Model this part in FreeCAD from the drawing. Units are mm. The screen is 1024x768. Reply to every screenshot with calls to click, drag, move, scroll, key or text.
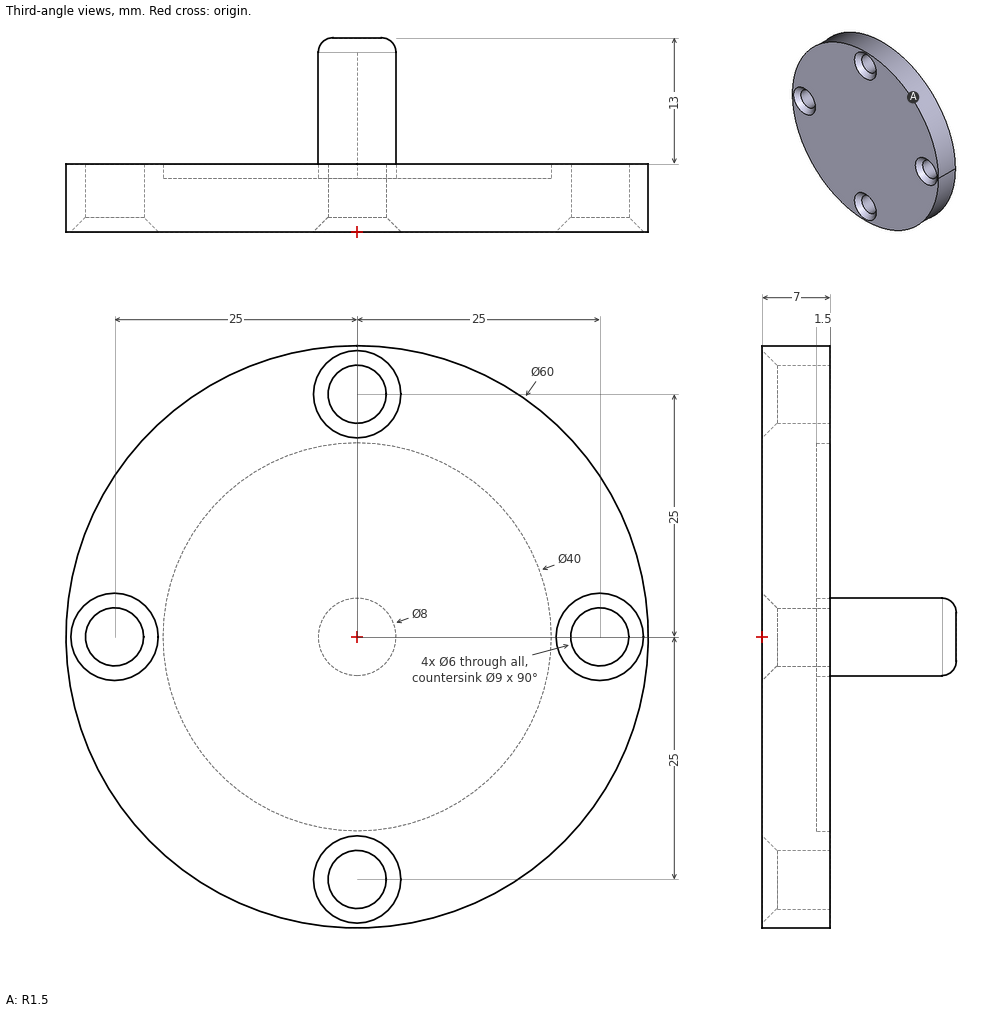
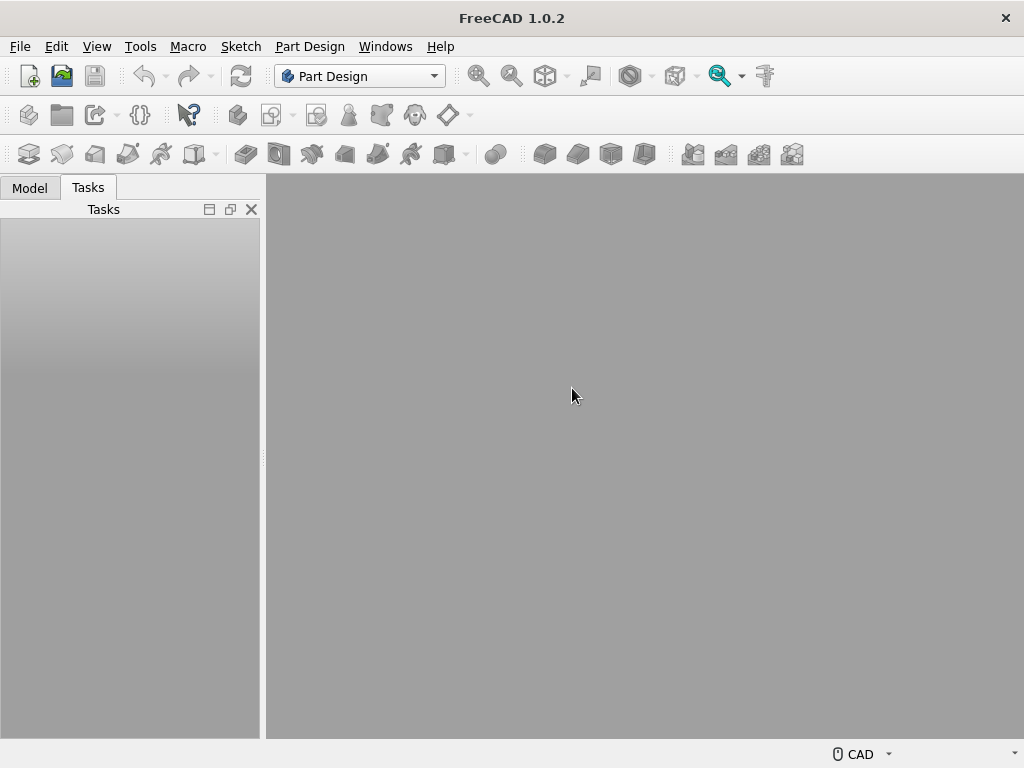
click(29, 76)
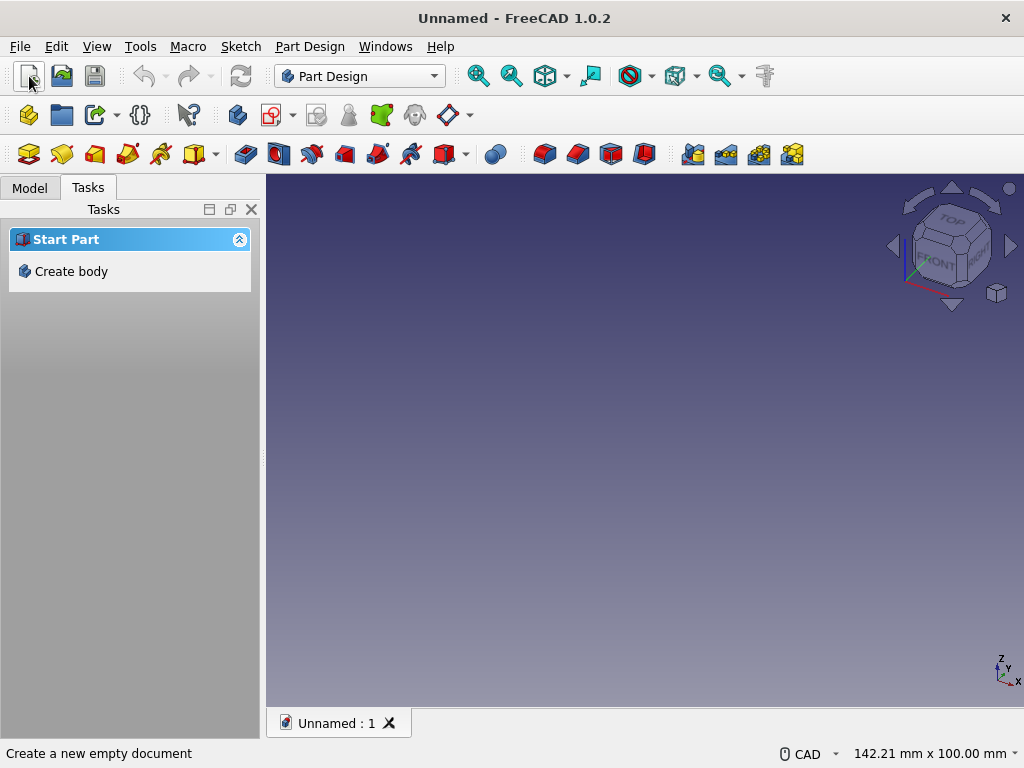
click(270, 116)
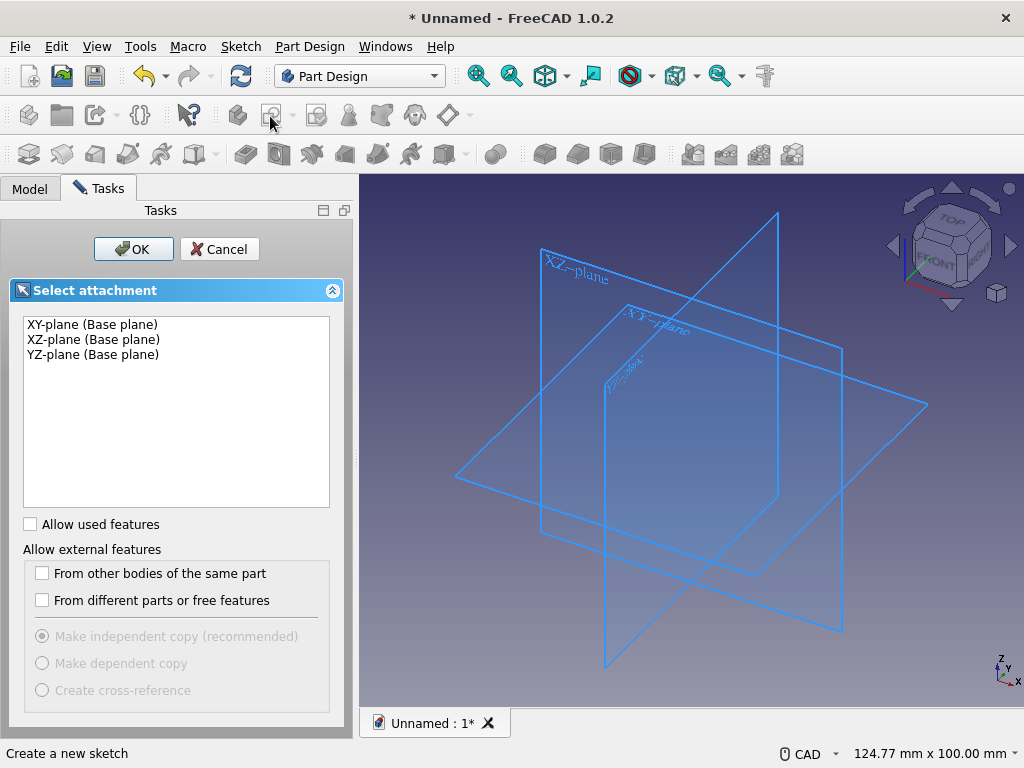
click(84, 340)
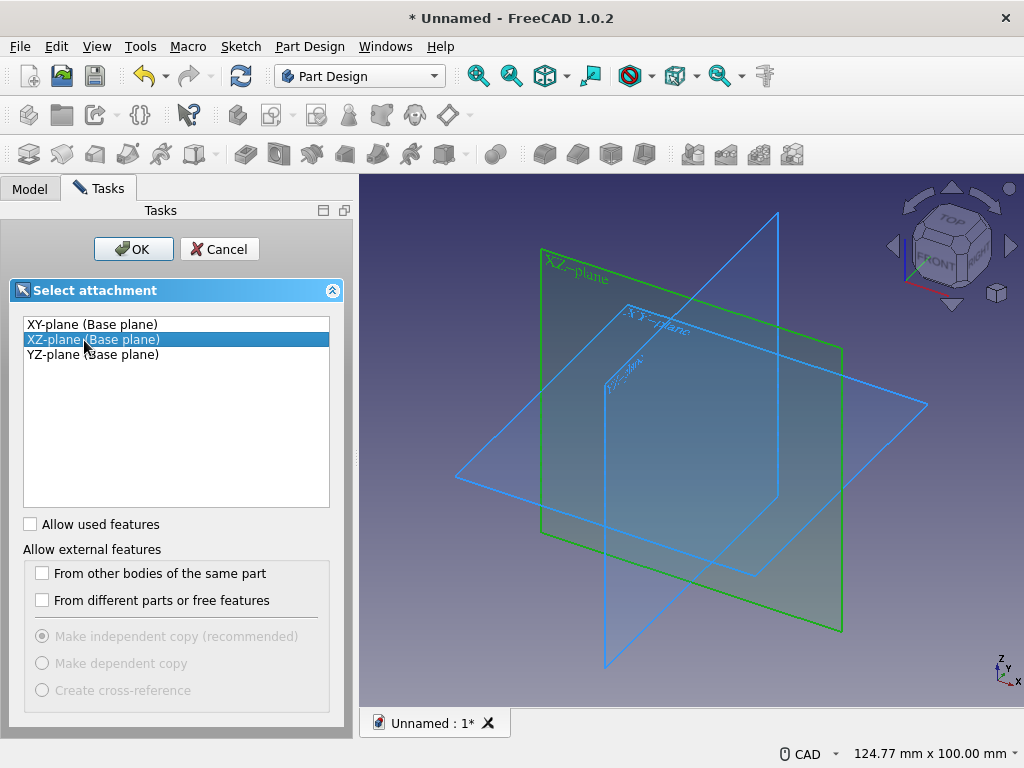
click(134, 249)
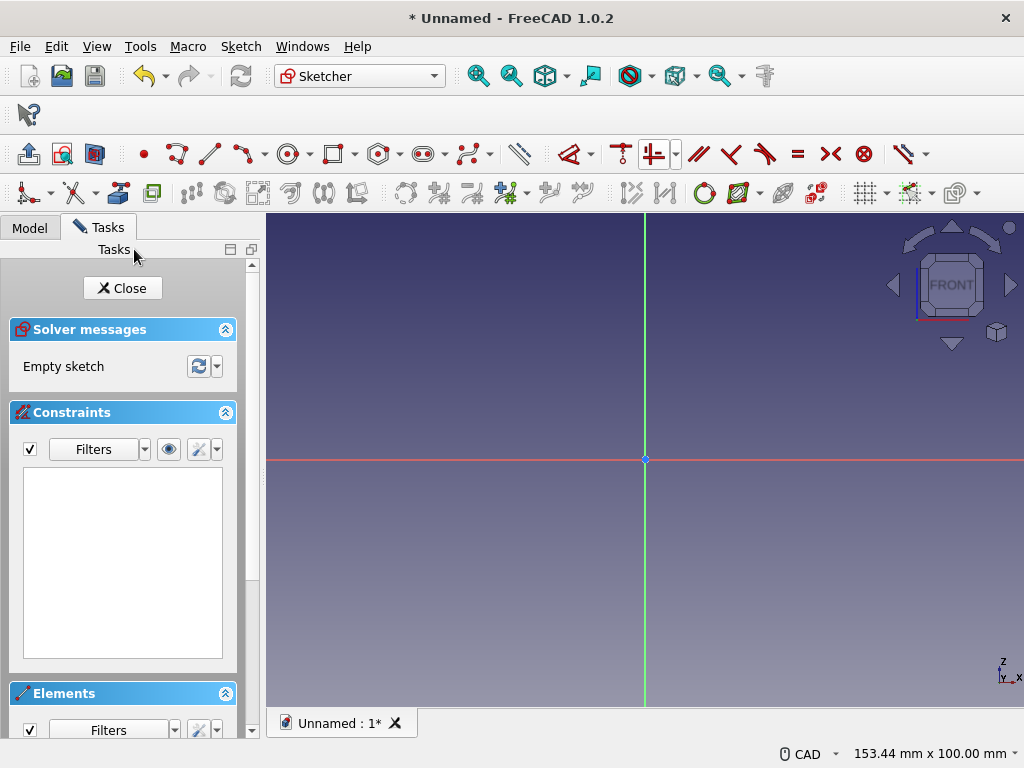
click(288, 154)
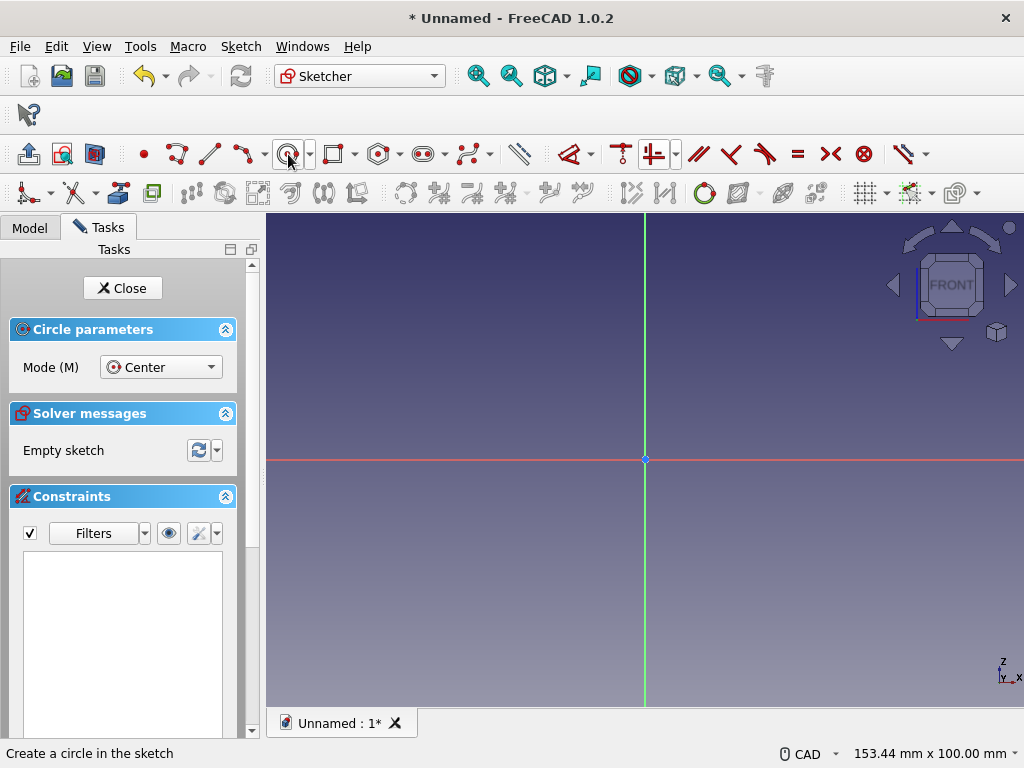
click(645, 460)
move(750, 355)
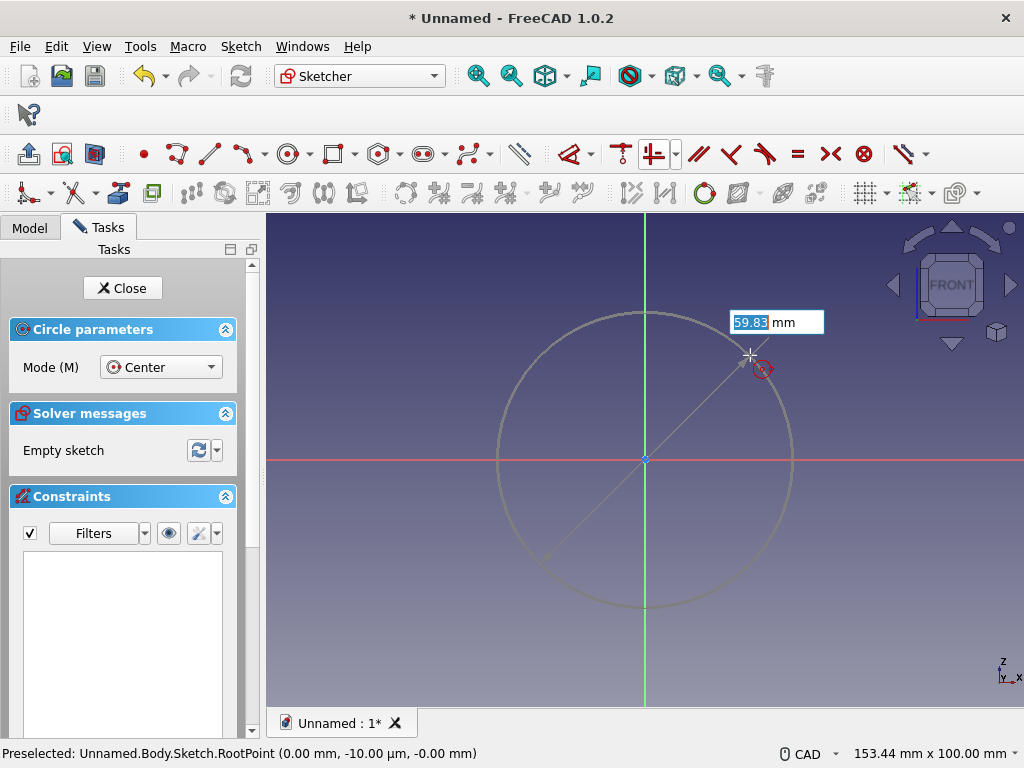
text(60)
key(Return)
key(Escape)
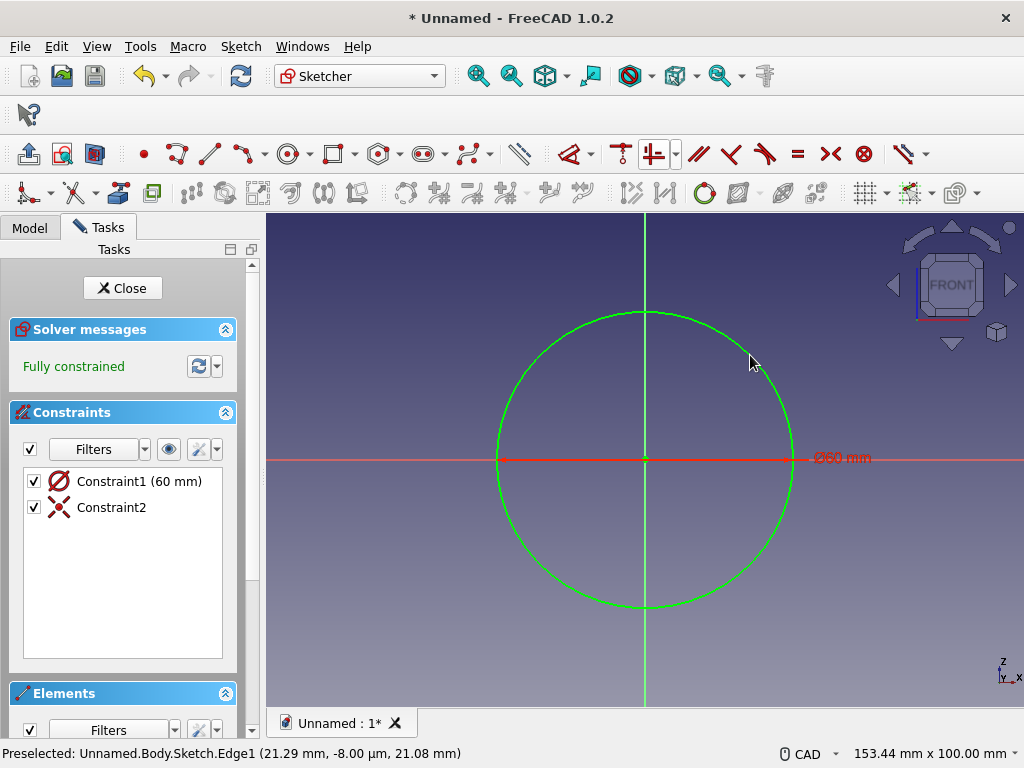
click(123, 288)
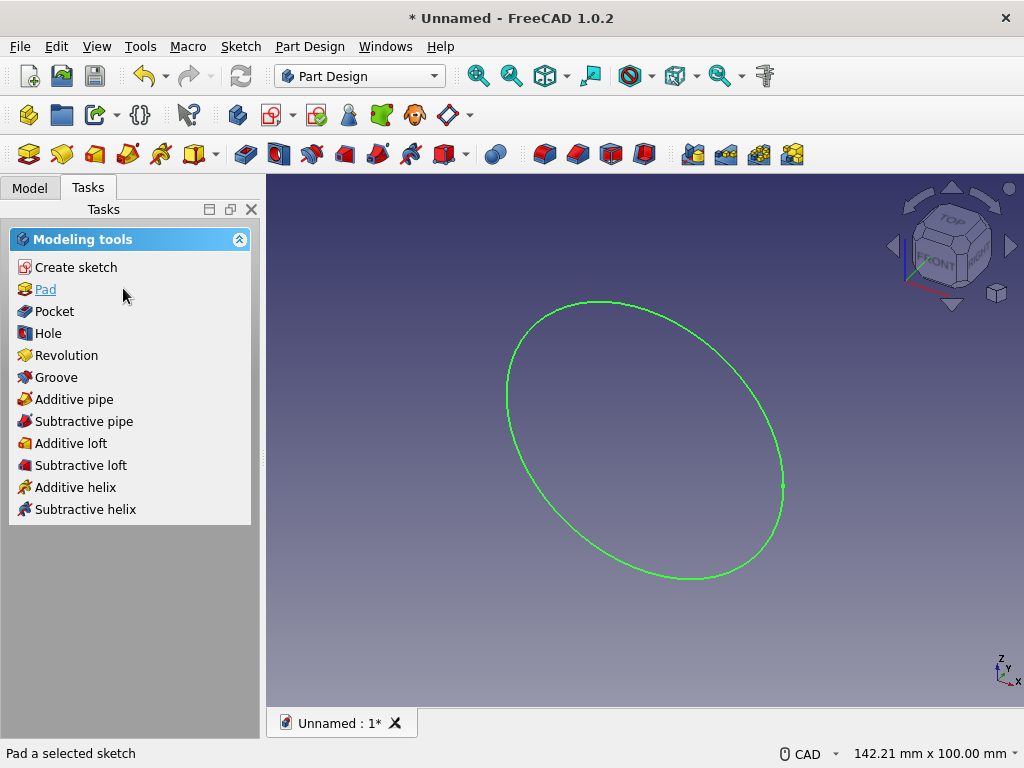
click(29, 154)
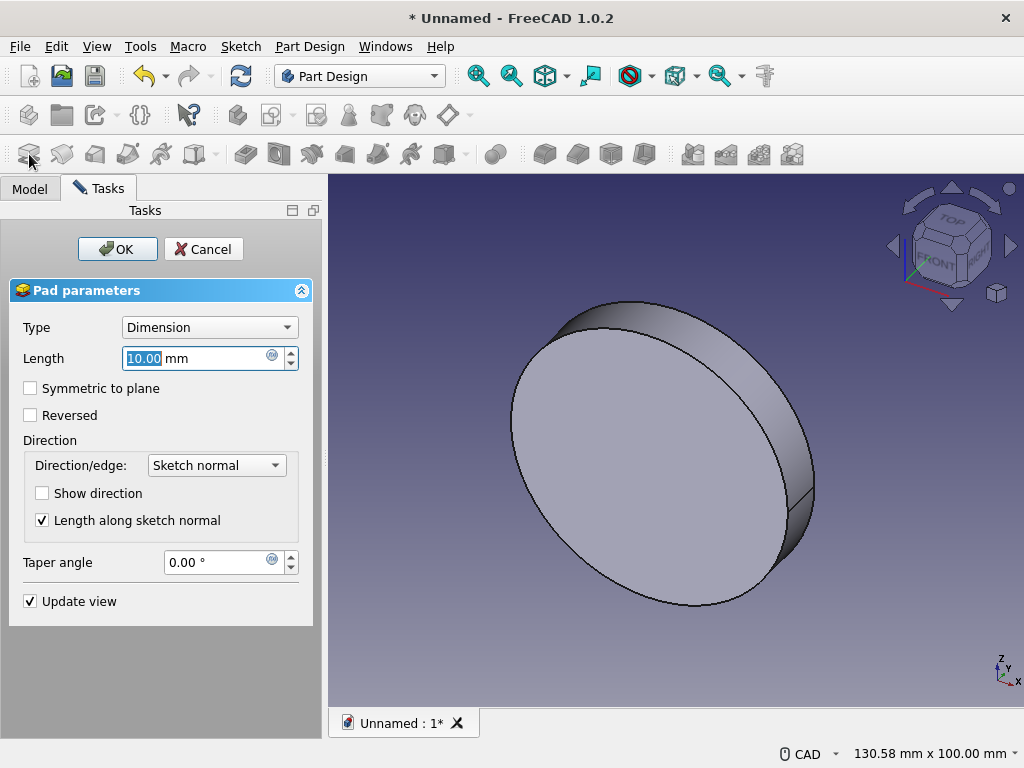
text(7)
key(Tab)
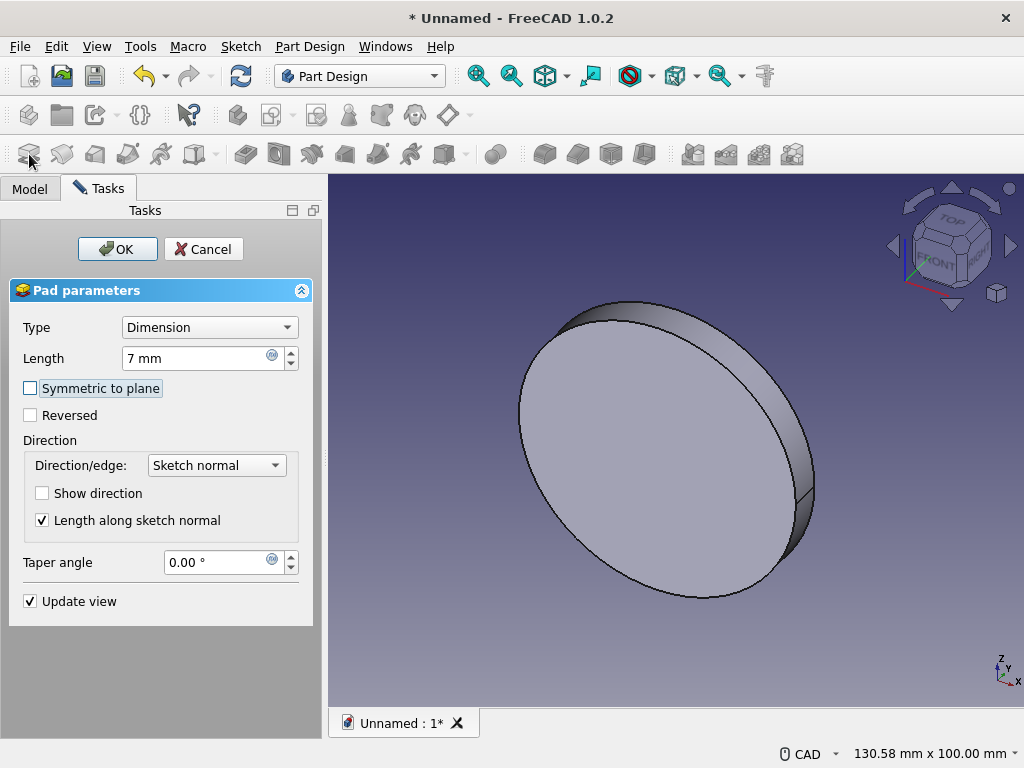
click(31, 415)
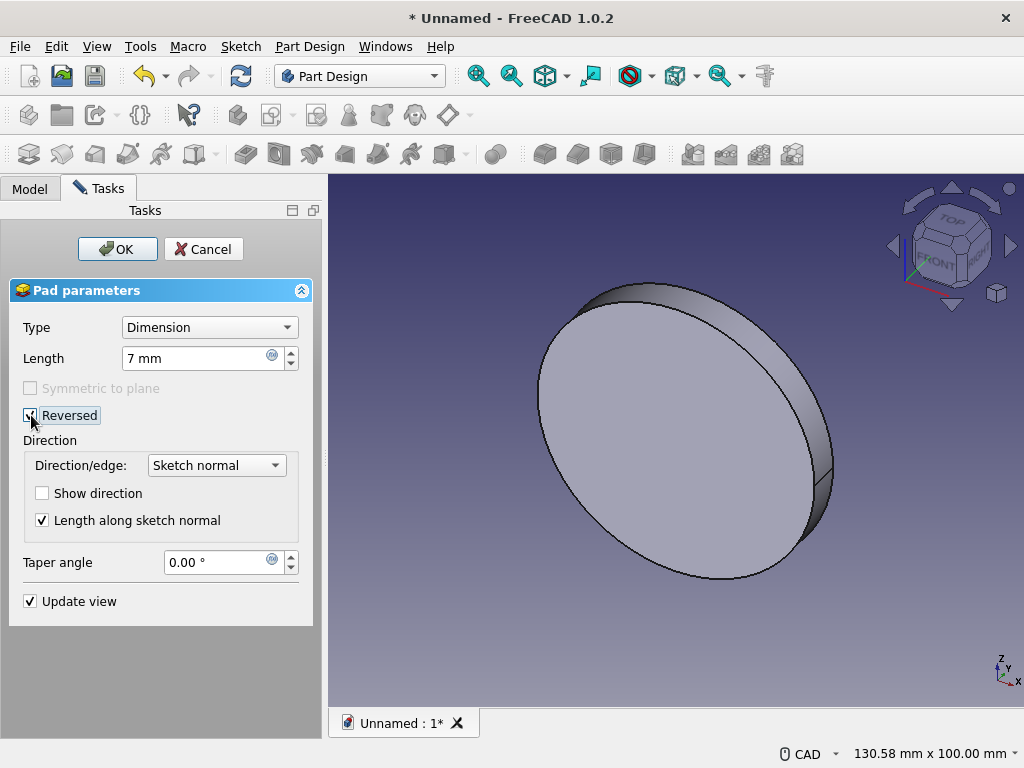
click(118, 249)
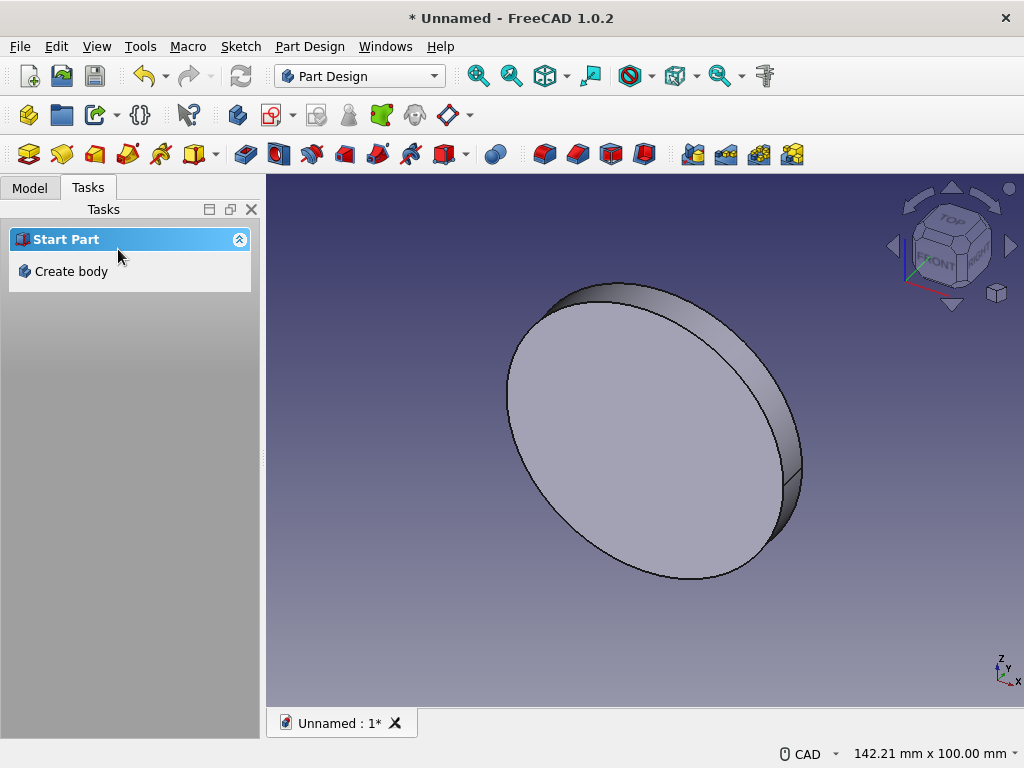
key(4)